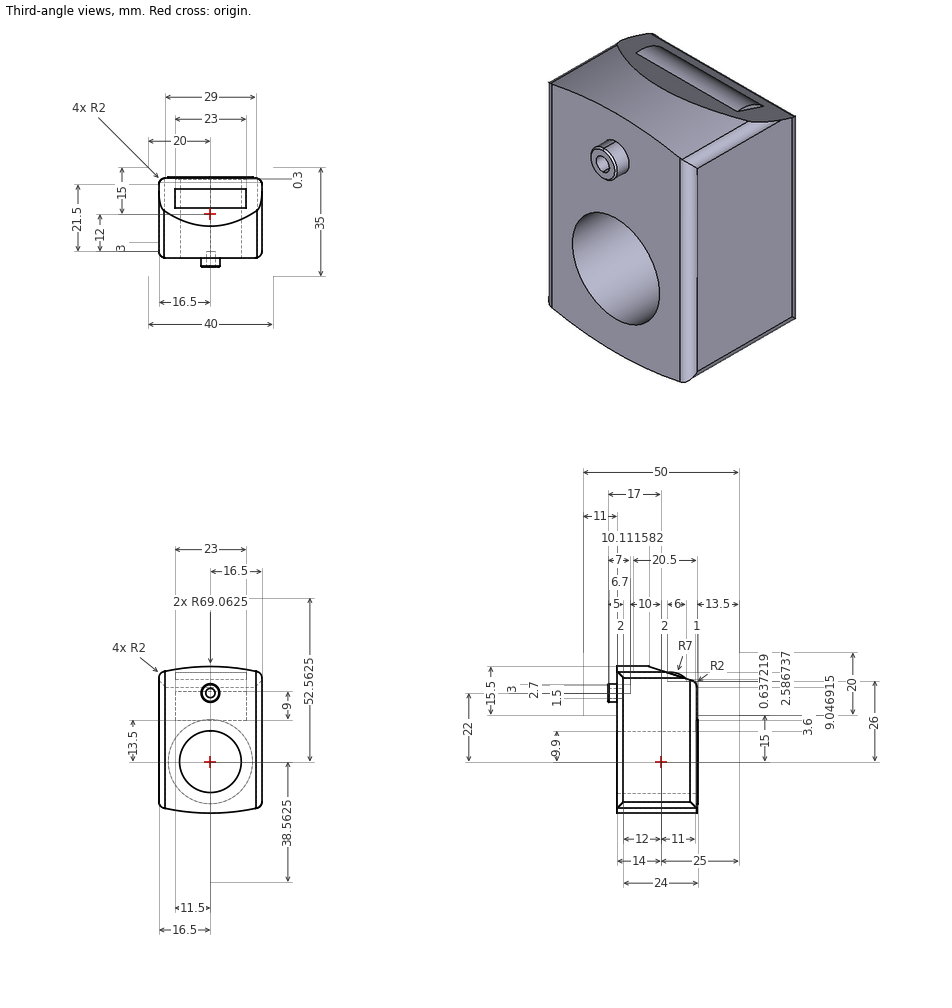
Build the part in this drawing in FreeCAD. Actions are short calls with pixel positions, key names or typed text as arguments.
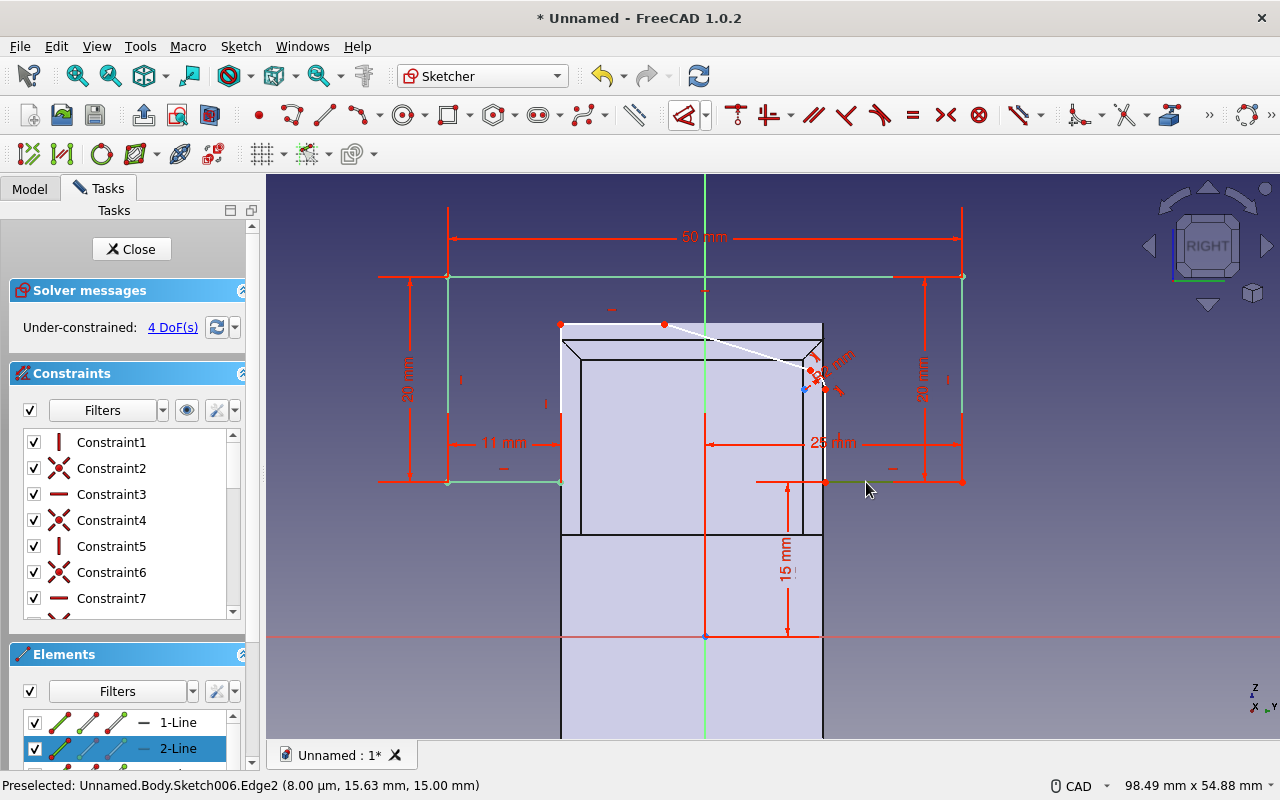
click(706, 116)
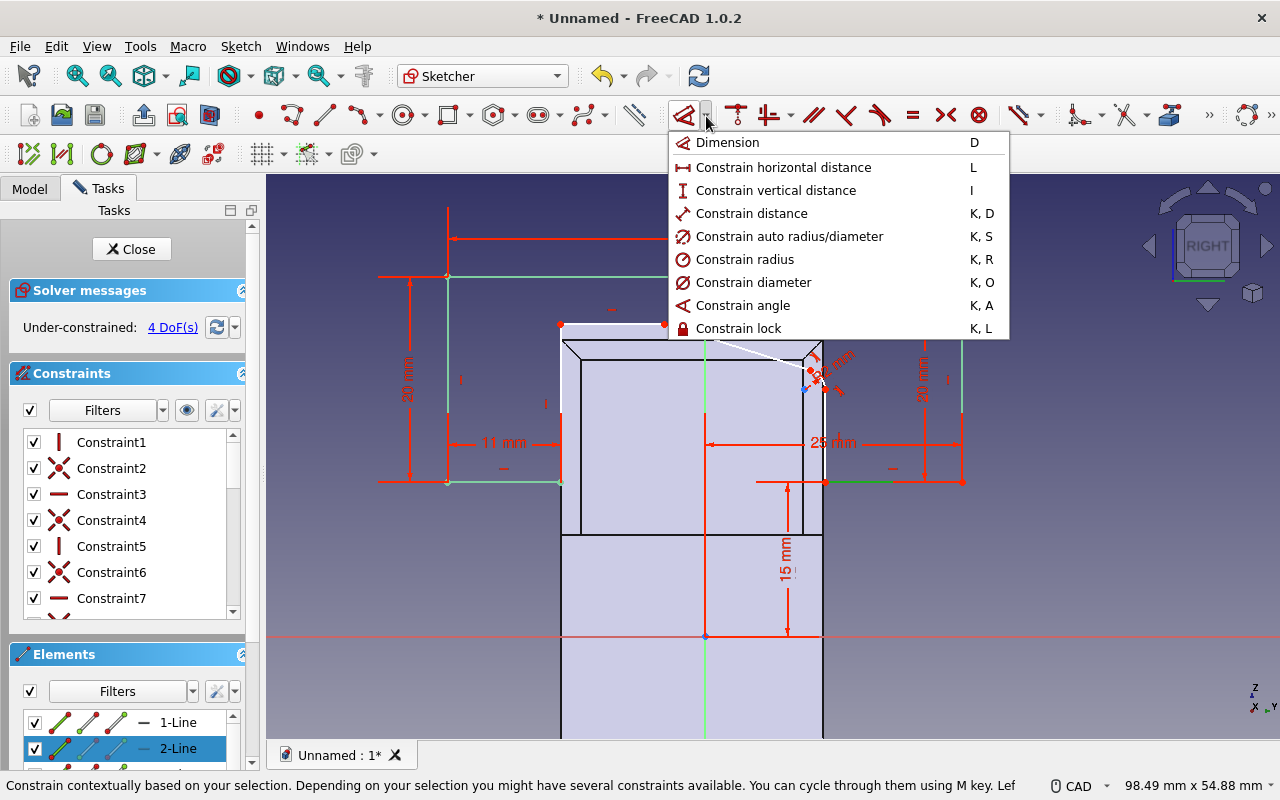
click(839, 168)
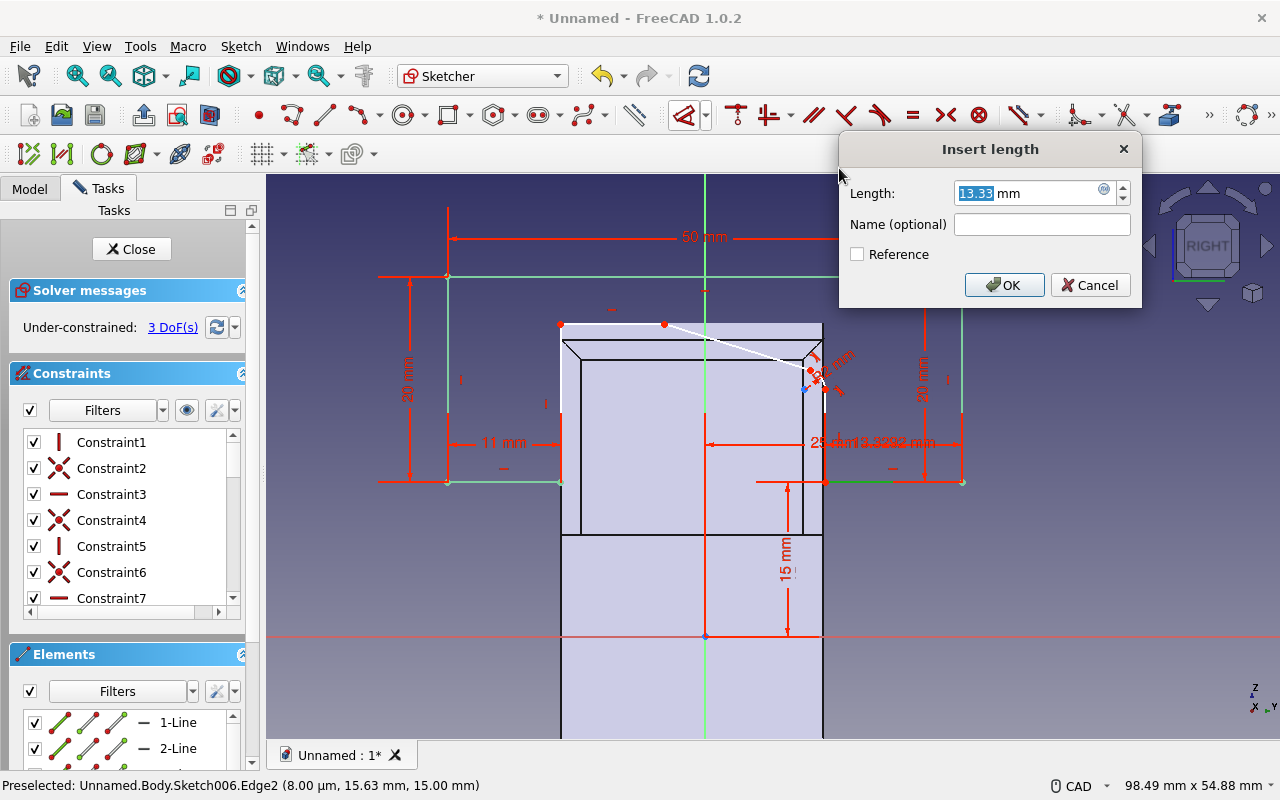
text(13.5)
key(Return)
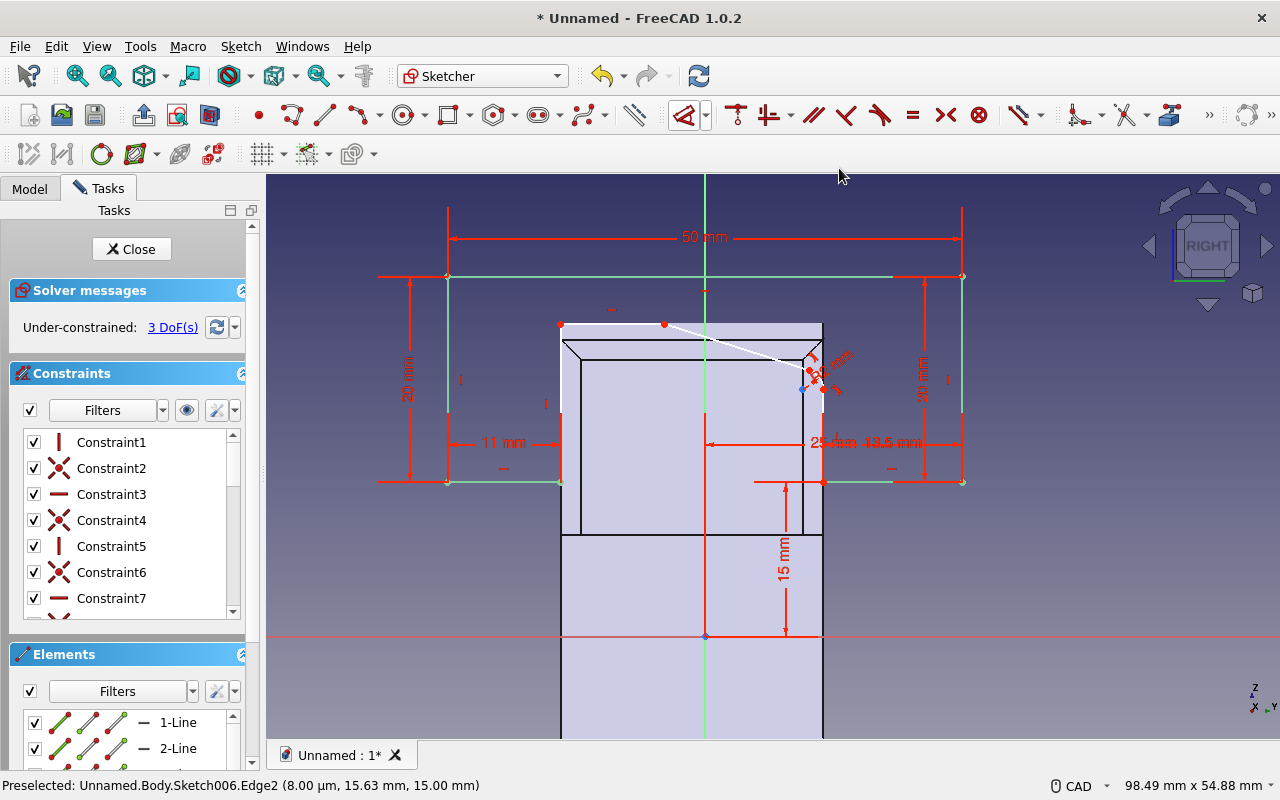
click(561, 435)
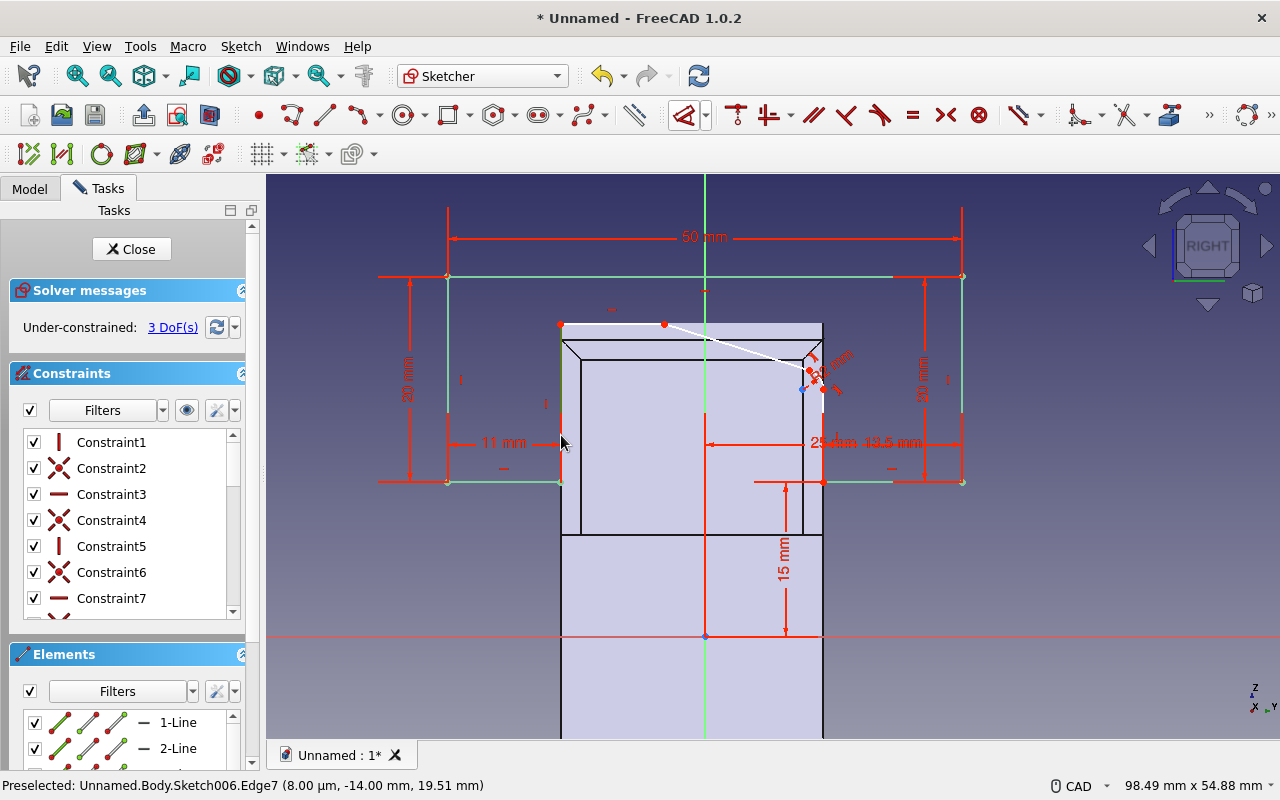
click(706, 116)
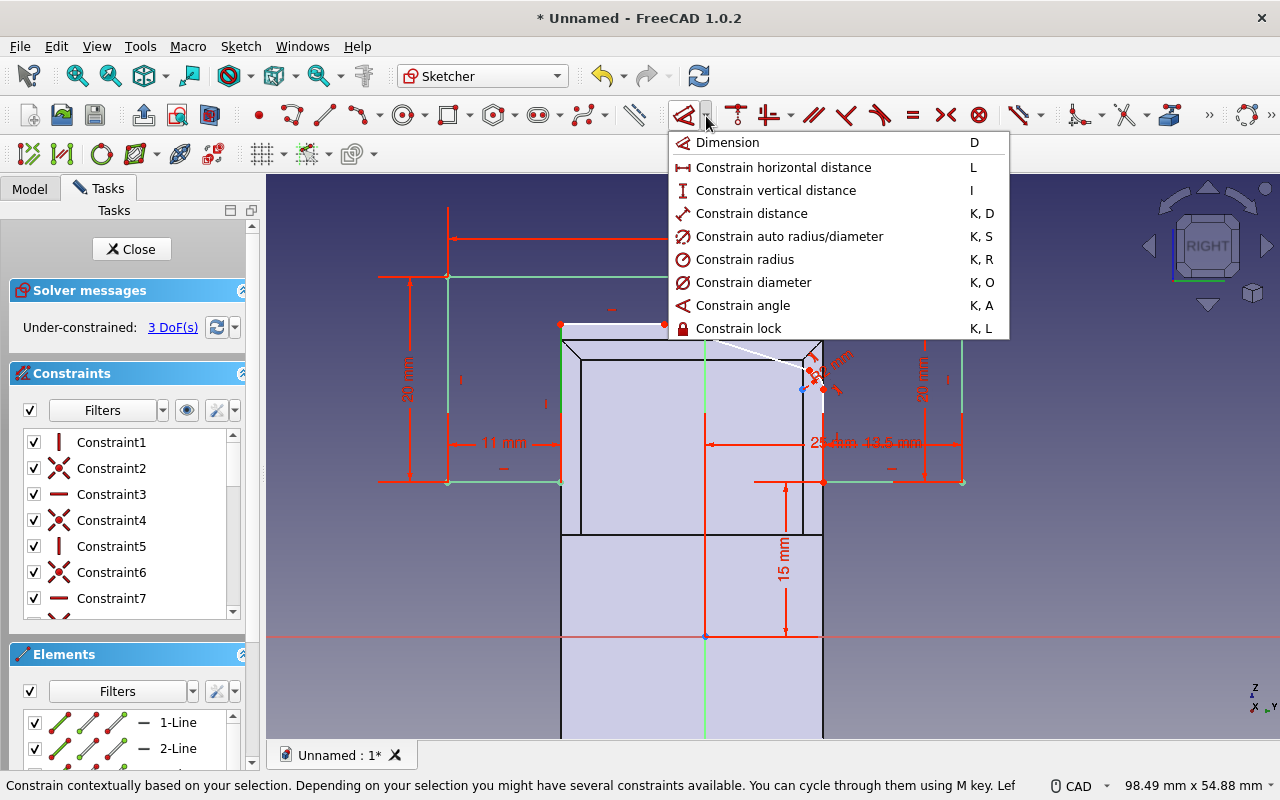
click(839, 190)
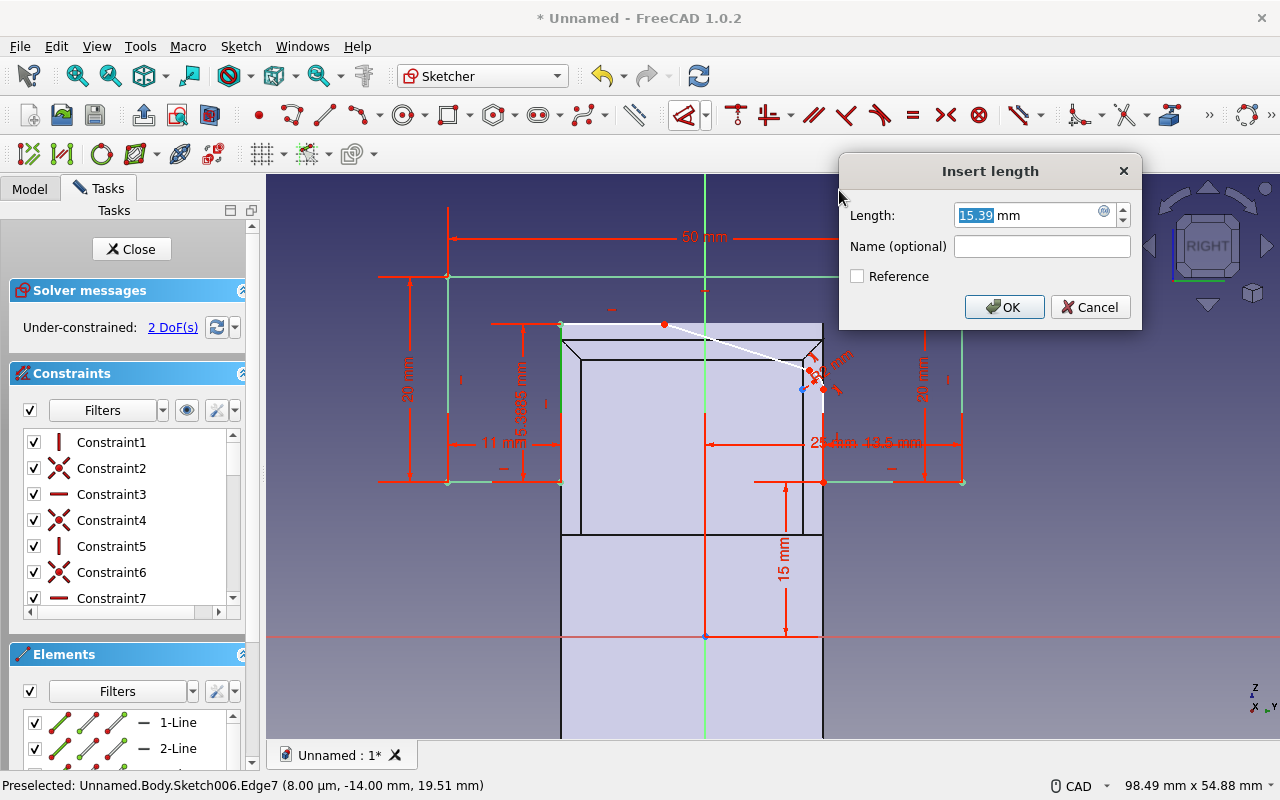
text(15.5)
key(Return)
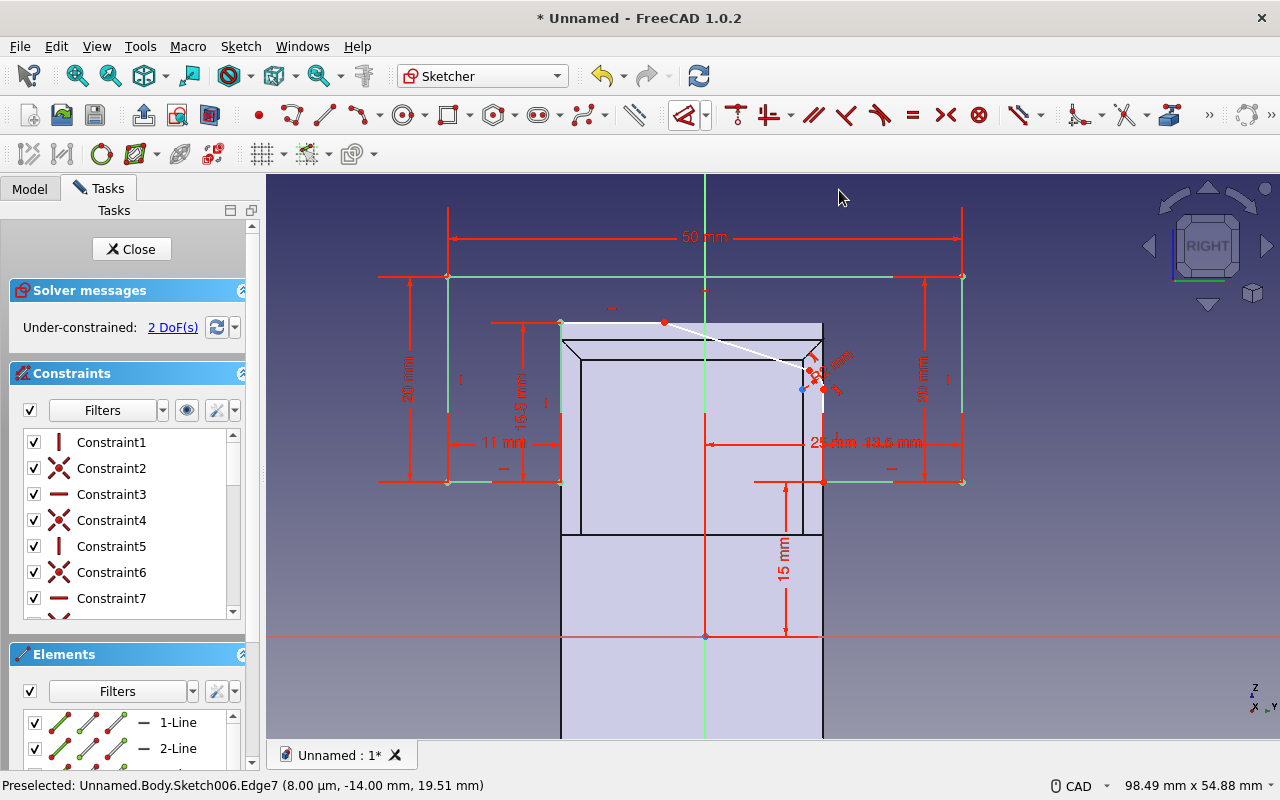
click(823, 418)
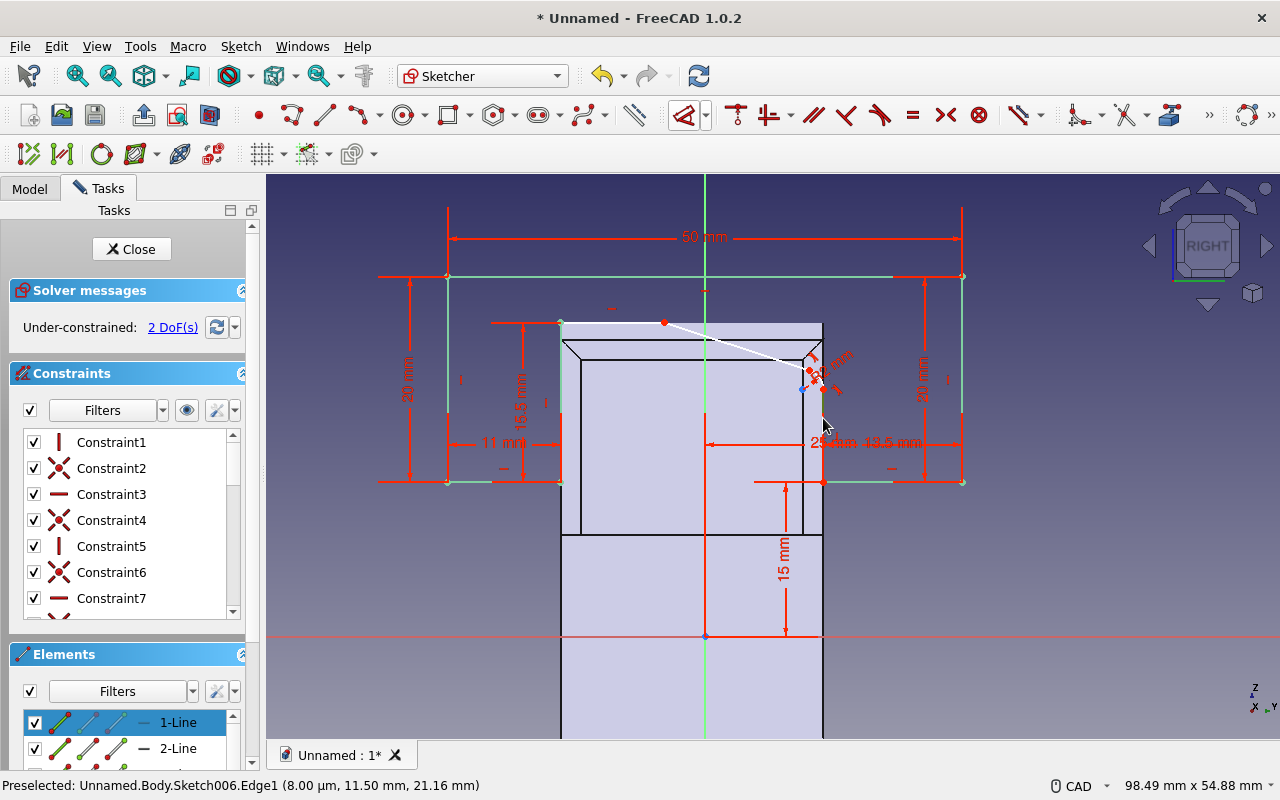
click(706, 116)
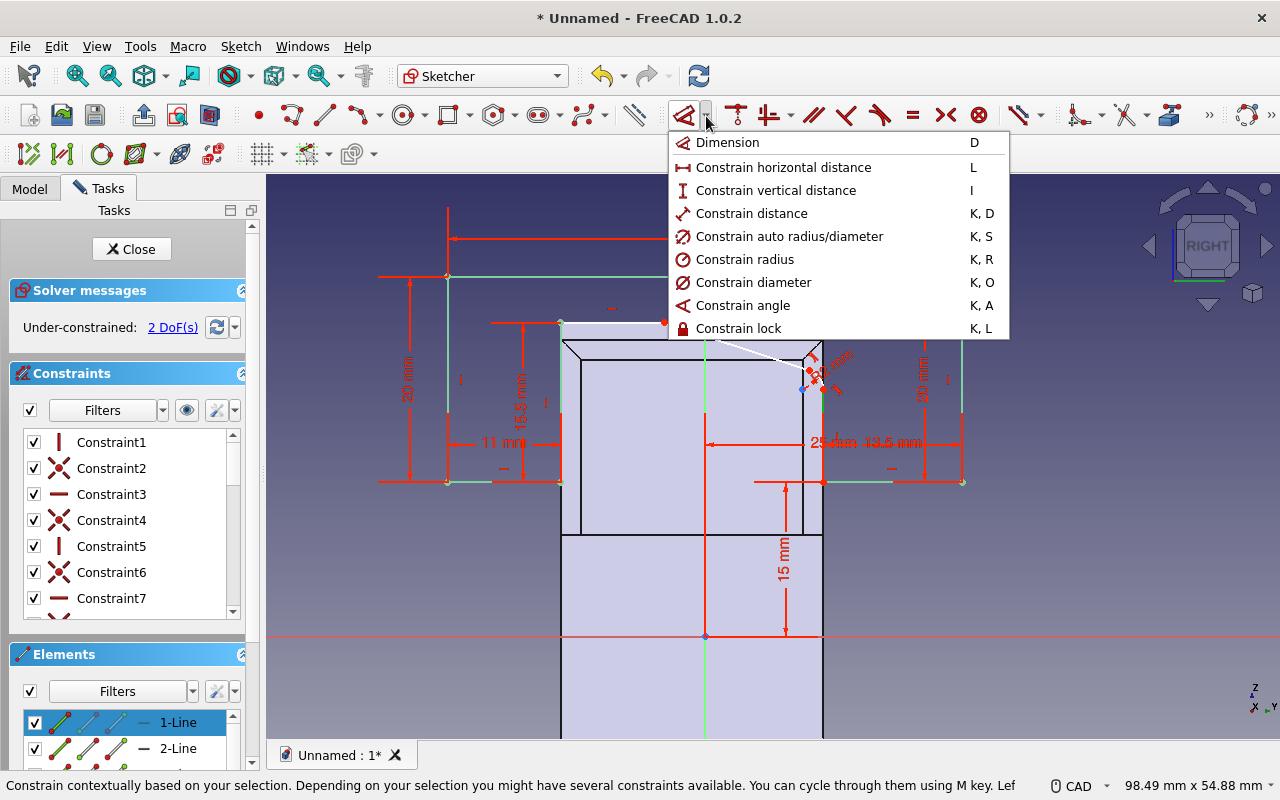
click(839, 190)